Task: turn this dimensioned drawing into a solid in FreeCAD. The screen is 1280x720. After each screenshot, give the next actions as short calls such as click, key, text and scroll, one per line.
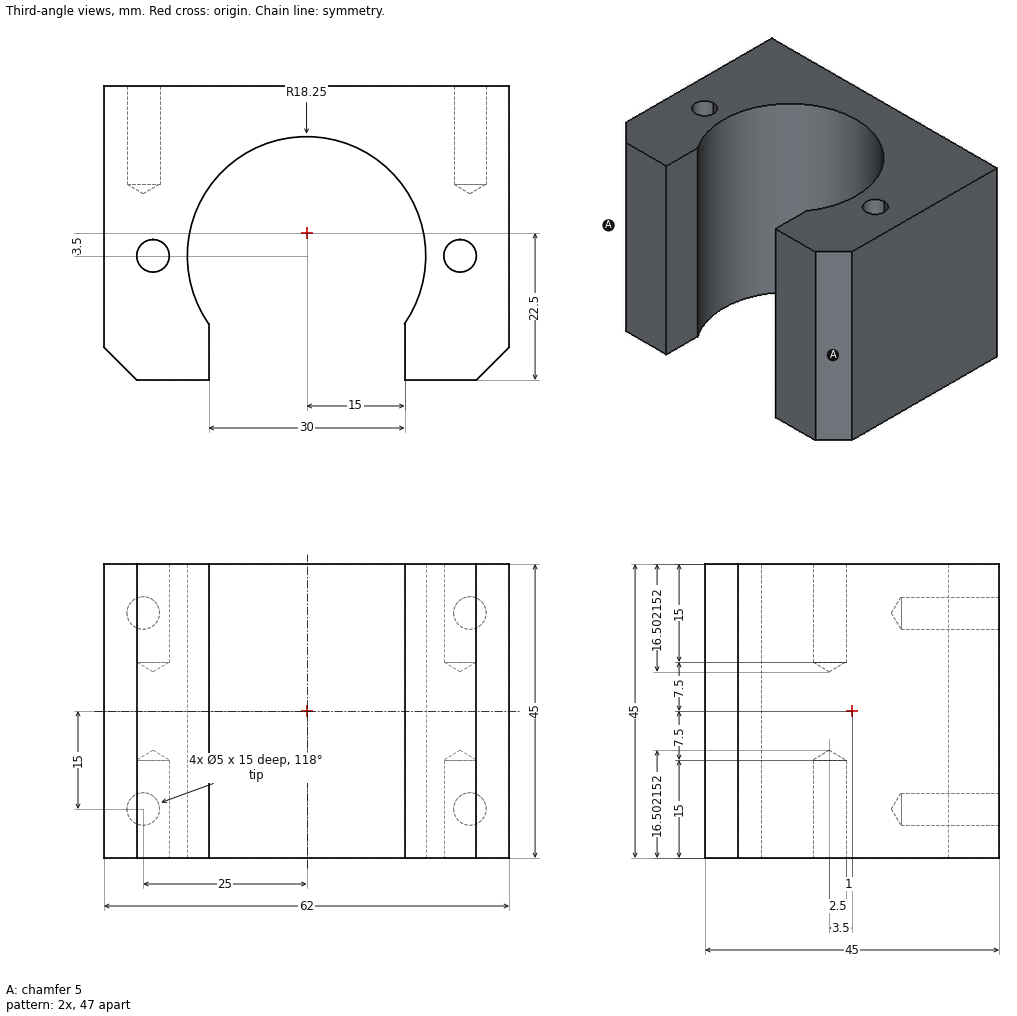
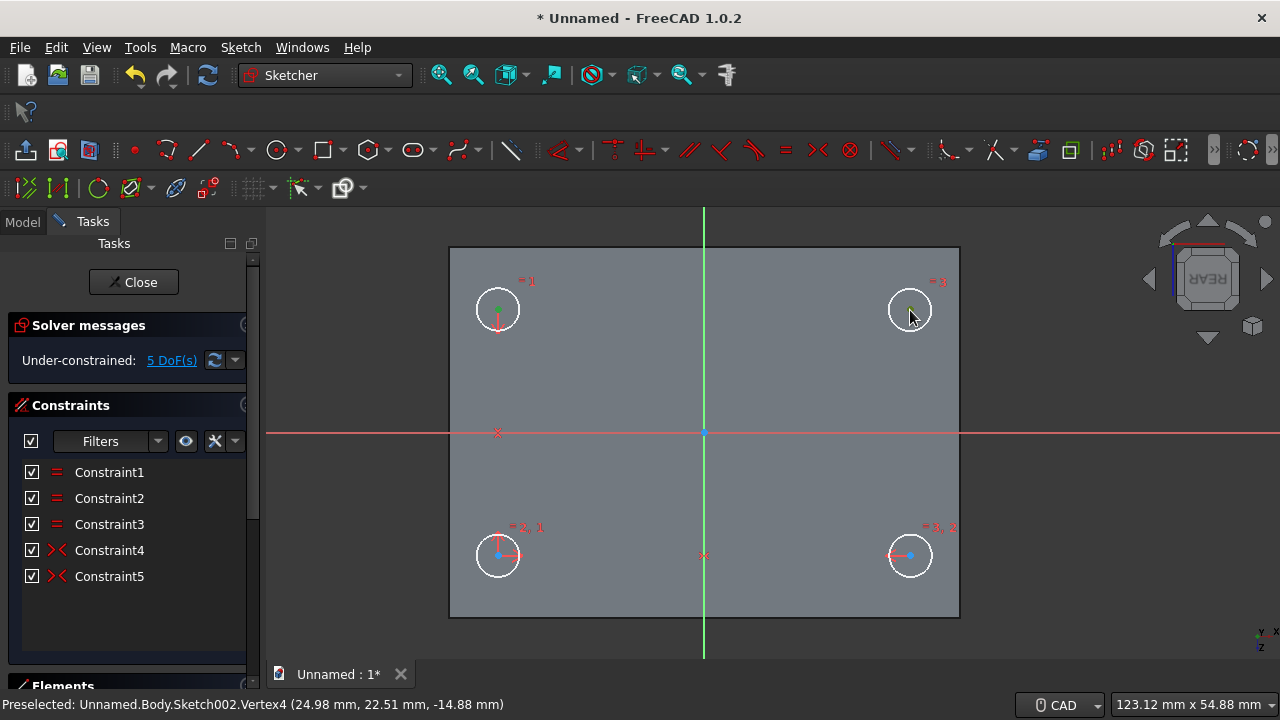
click(704, 603)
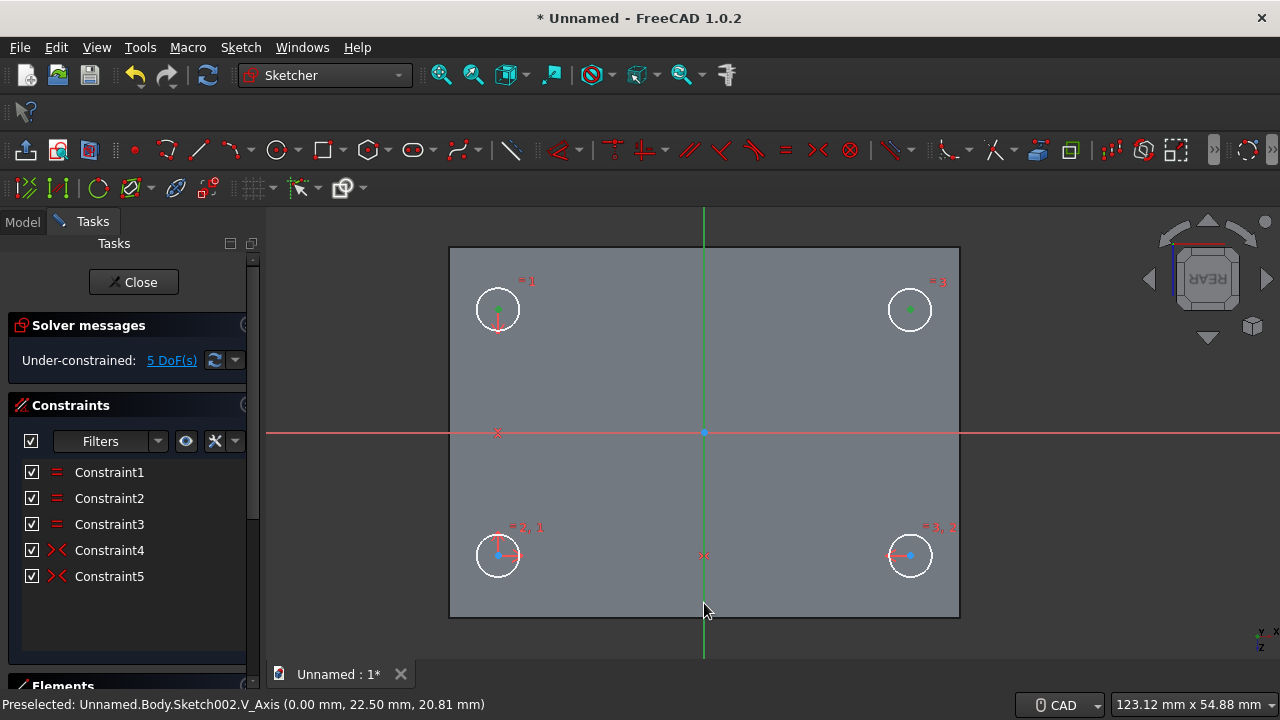
click(818, 150)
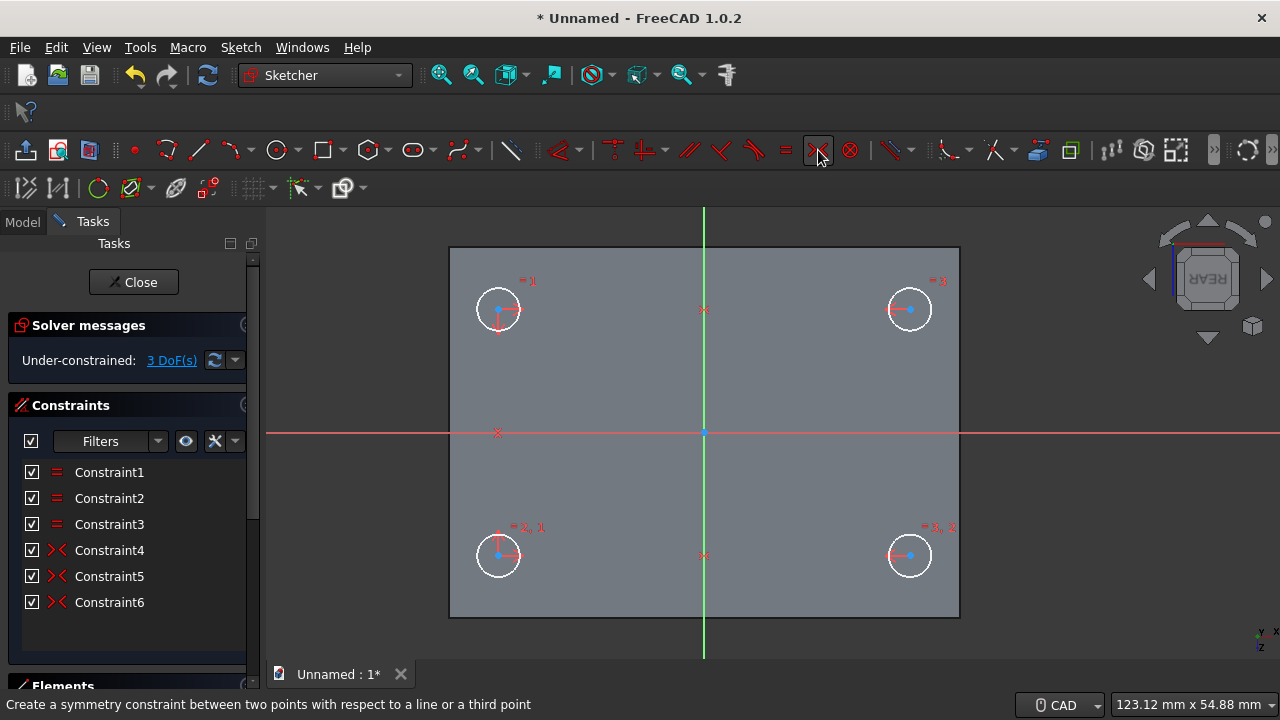
click(558, 150)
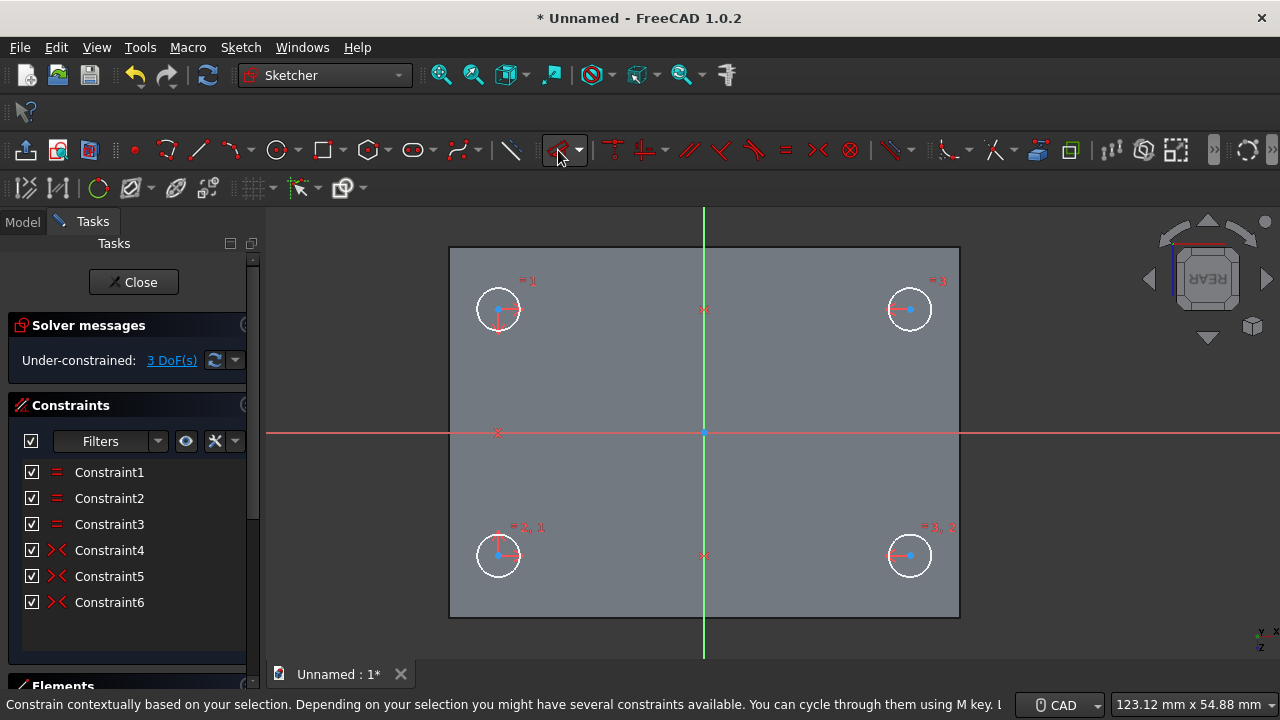
click(513, 294)
click(535, 271)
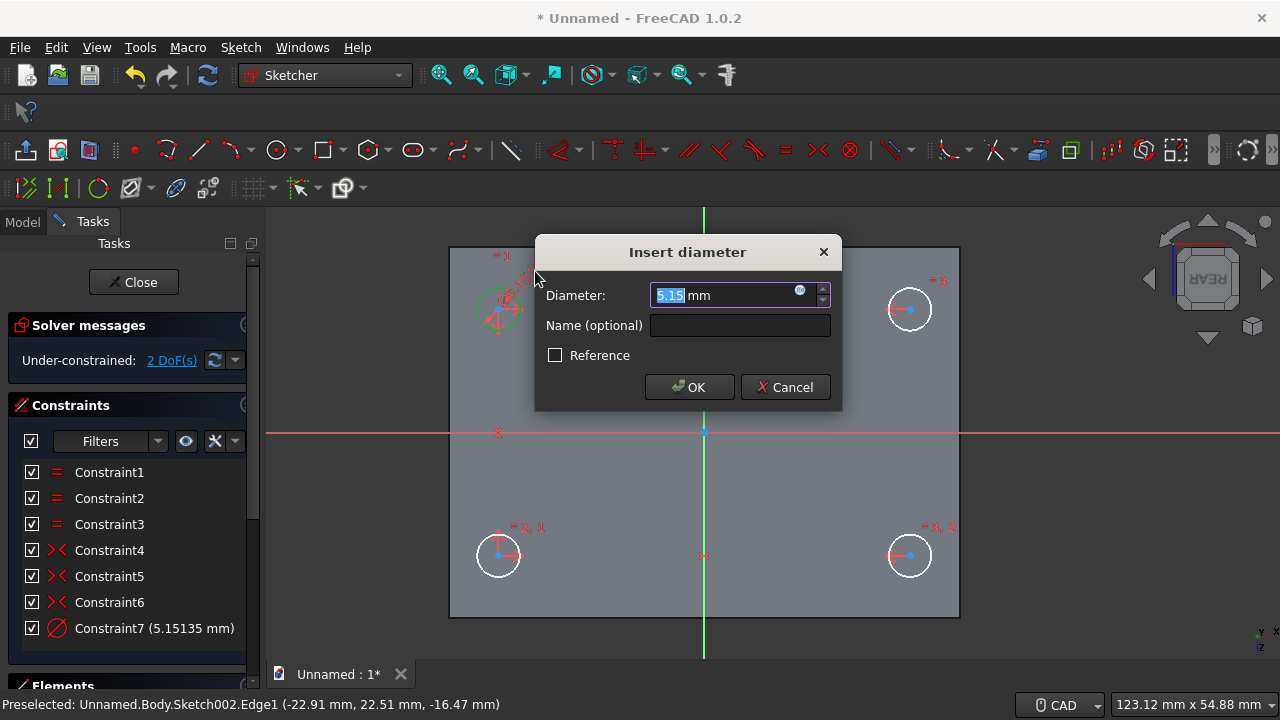
text(5)
key(Return)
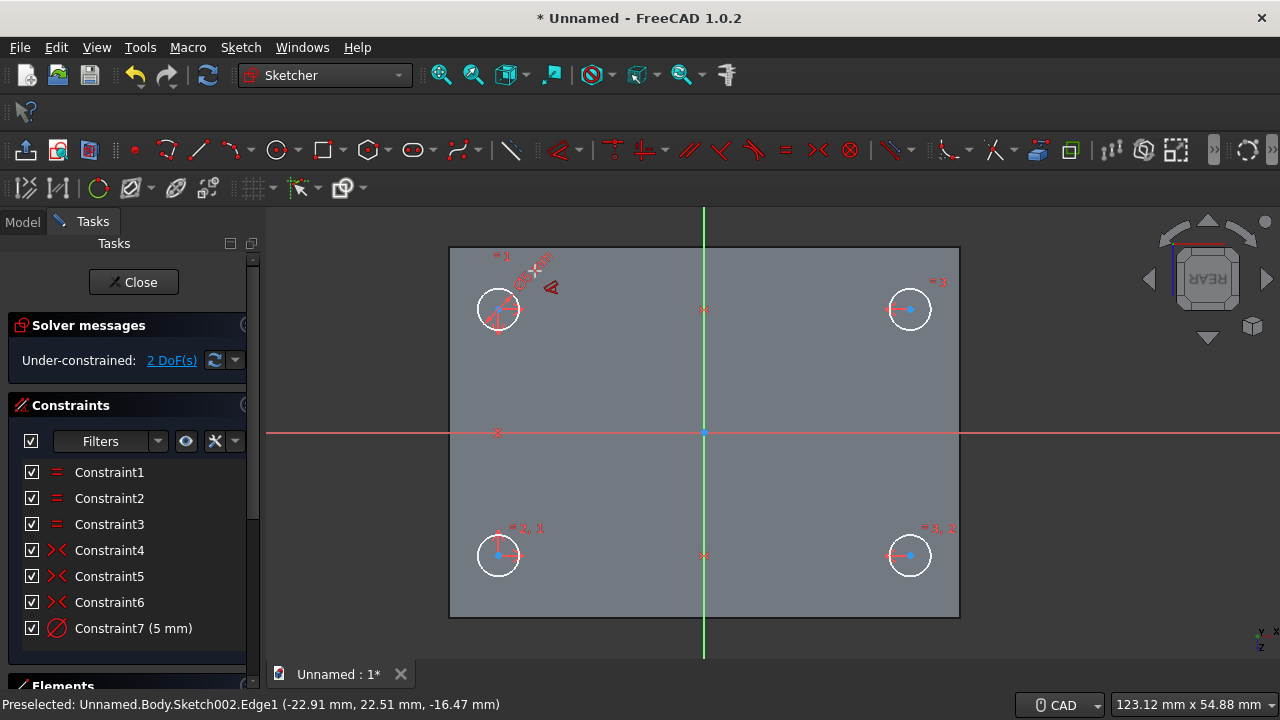
click(498, 309)
click(649, 275)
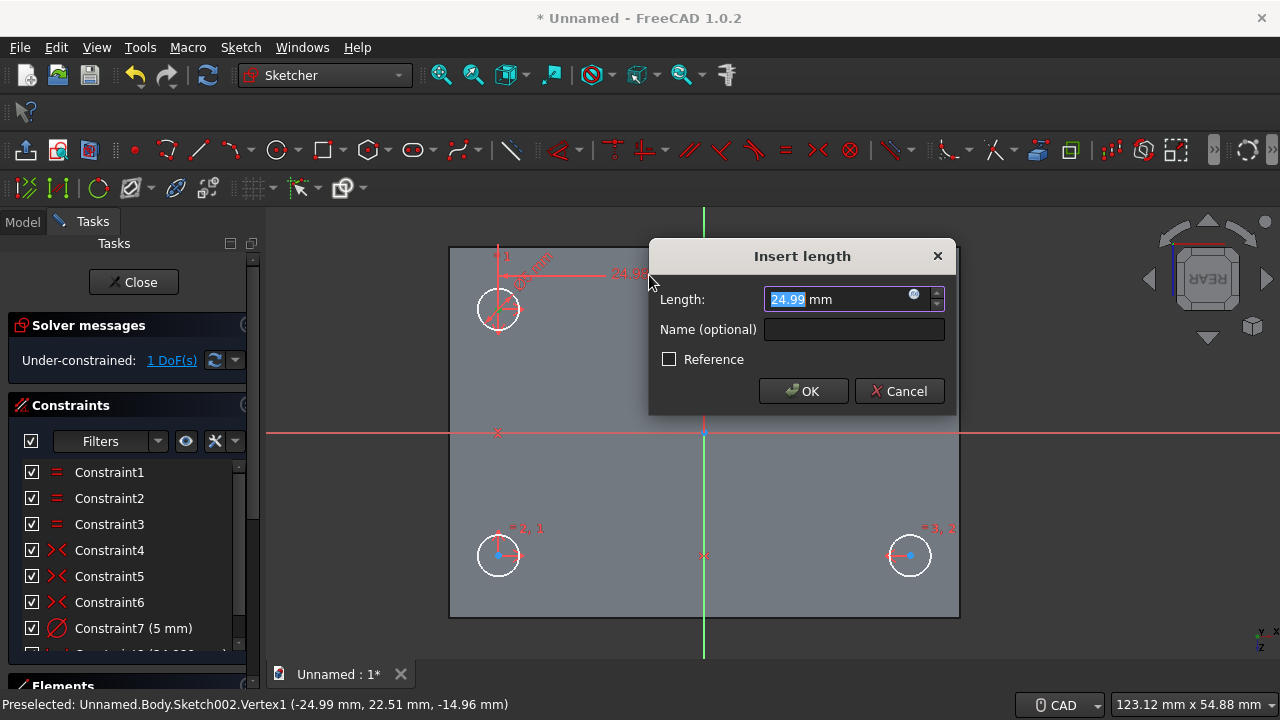
text(25)
key(Return)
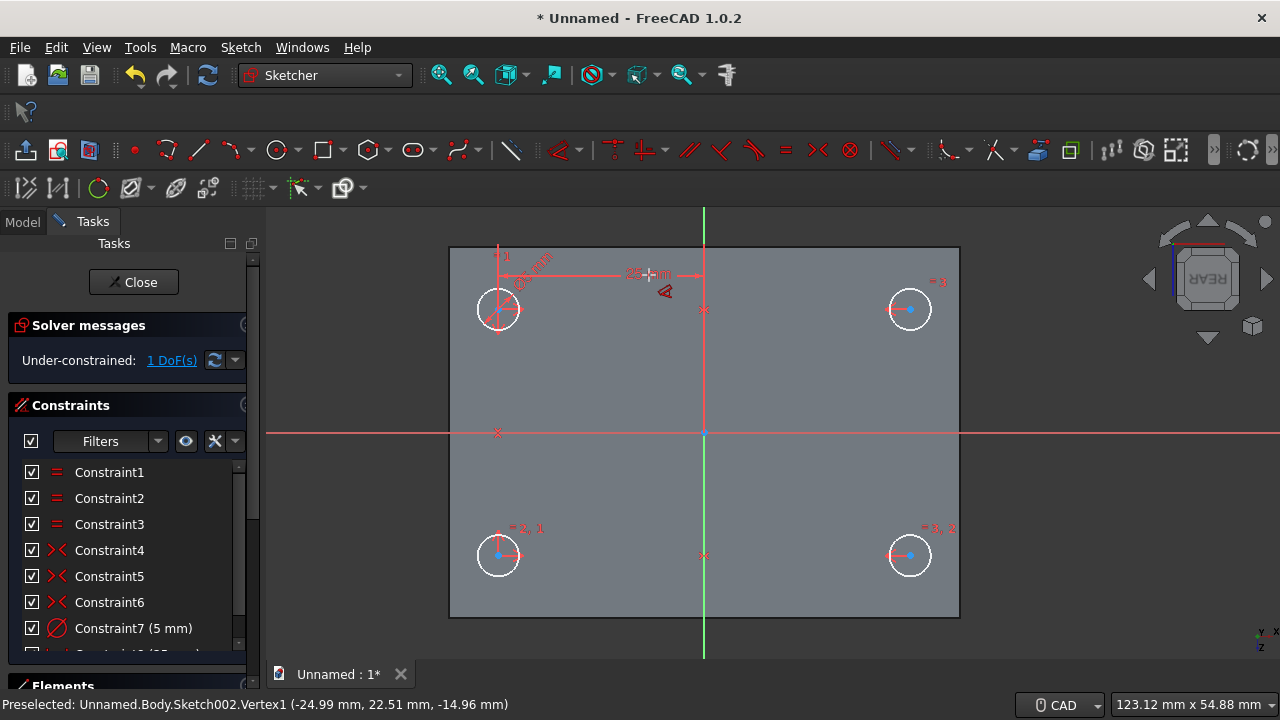
click(498, 309)
click(464, 371)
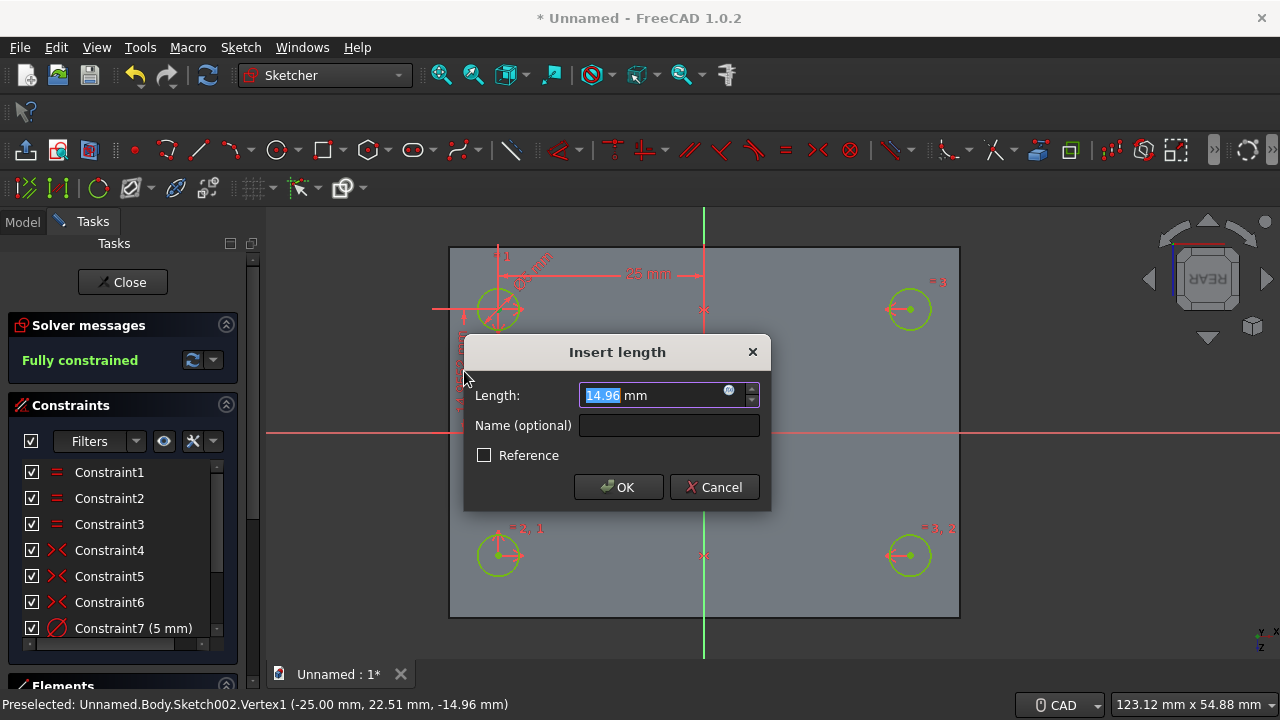
text(15)
key(Return)
key(Escape)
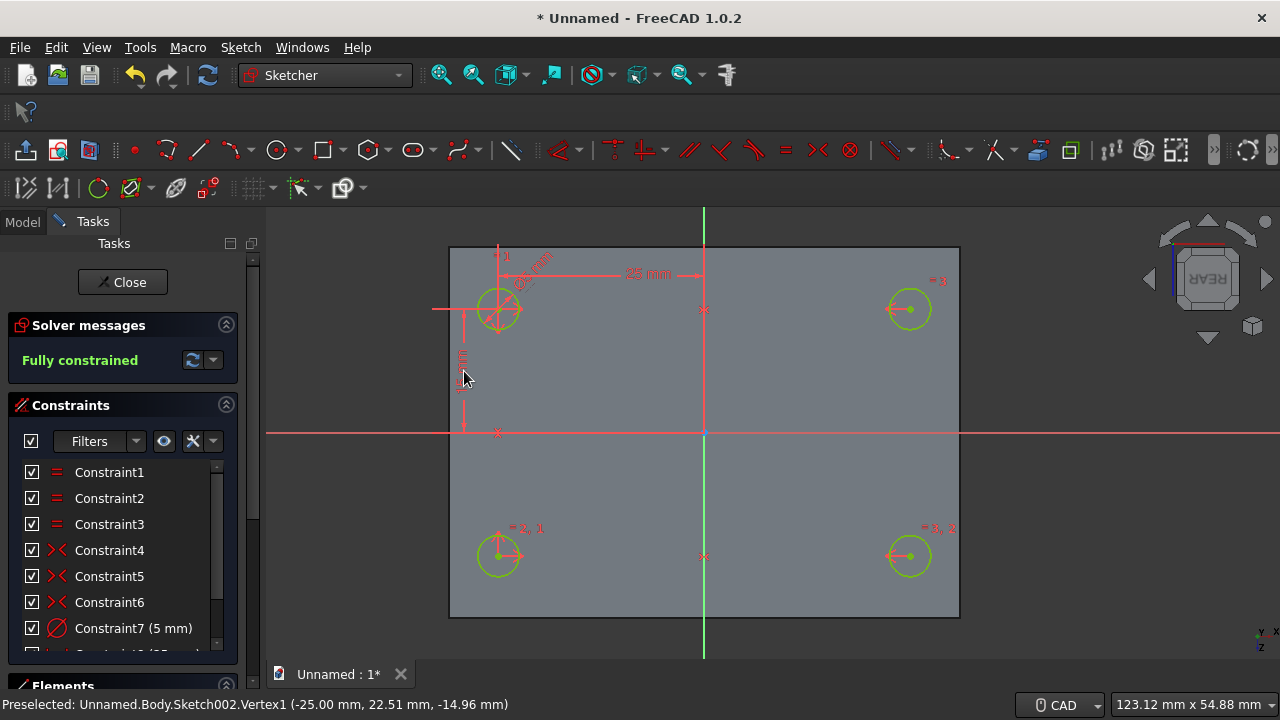
click(123, 282)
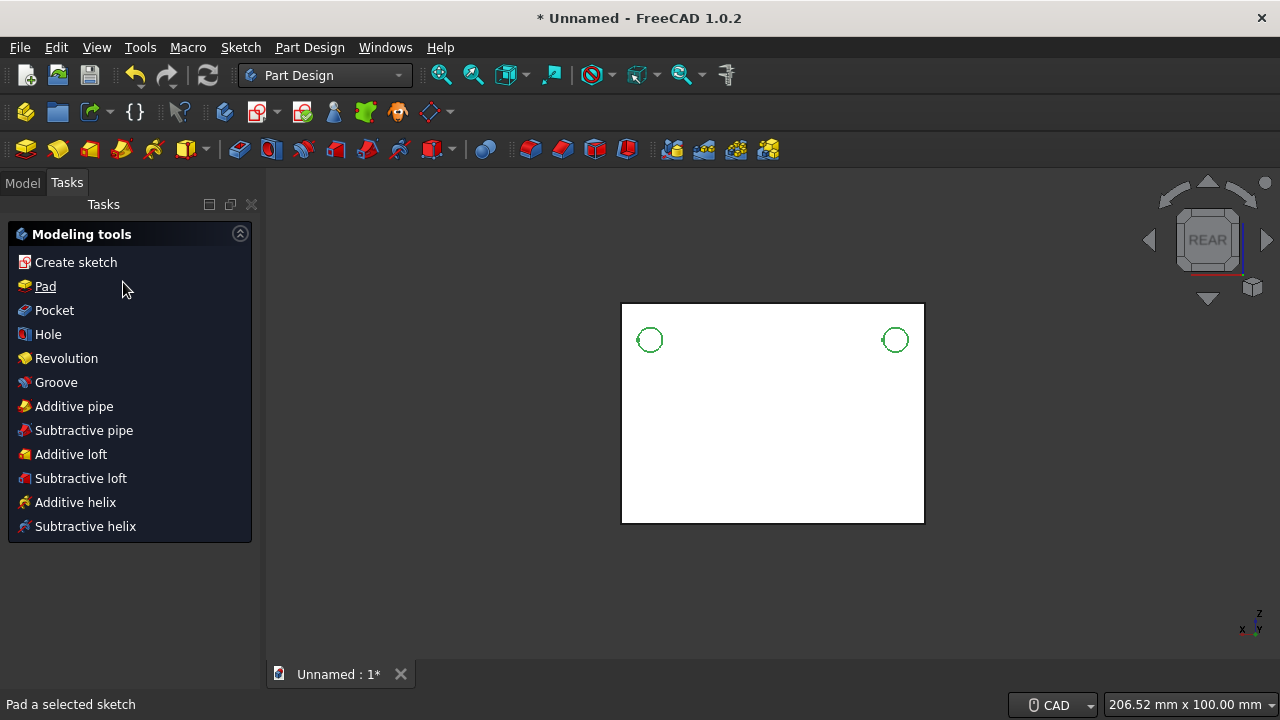
click(272, 150)